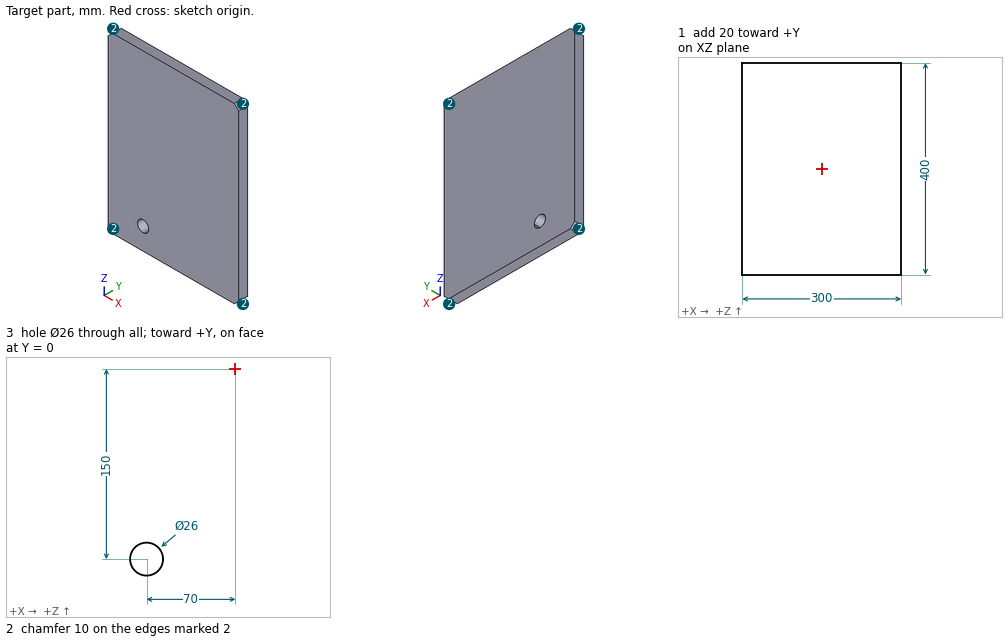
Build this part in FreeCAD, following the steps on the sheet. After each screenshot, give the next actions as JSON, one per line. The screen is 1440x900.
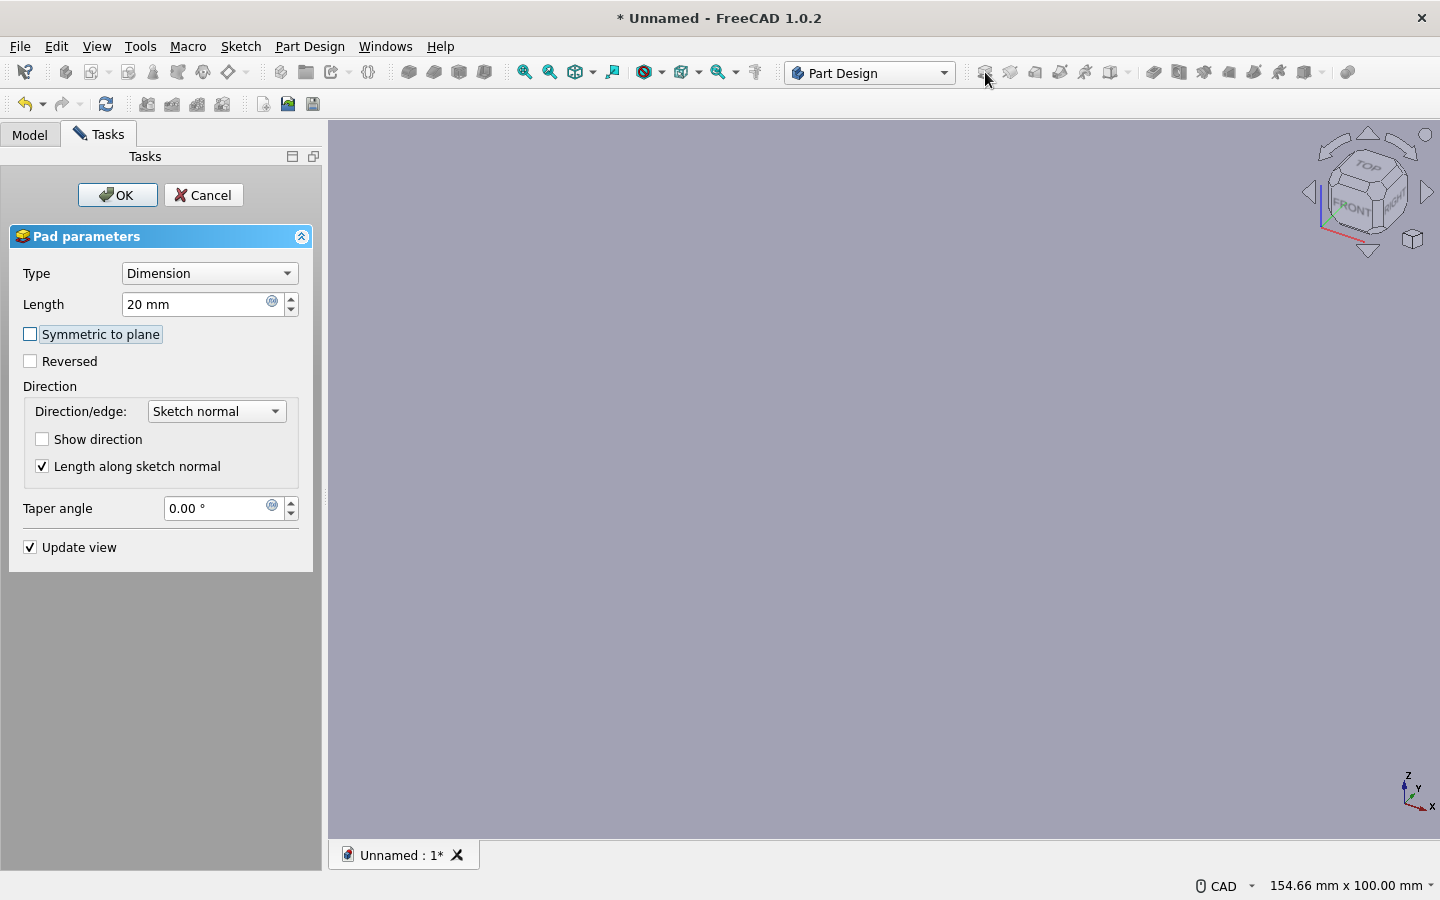
{"action": "left_click", "coordinate": [31, 361]}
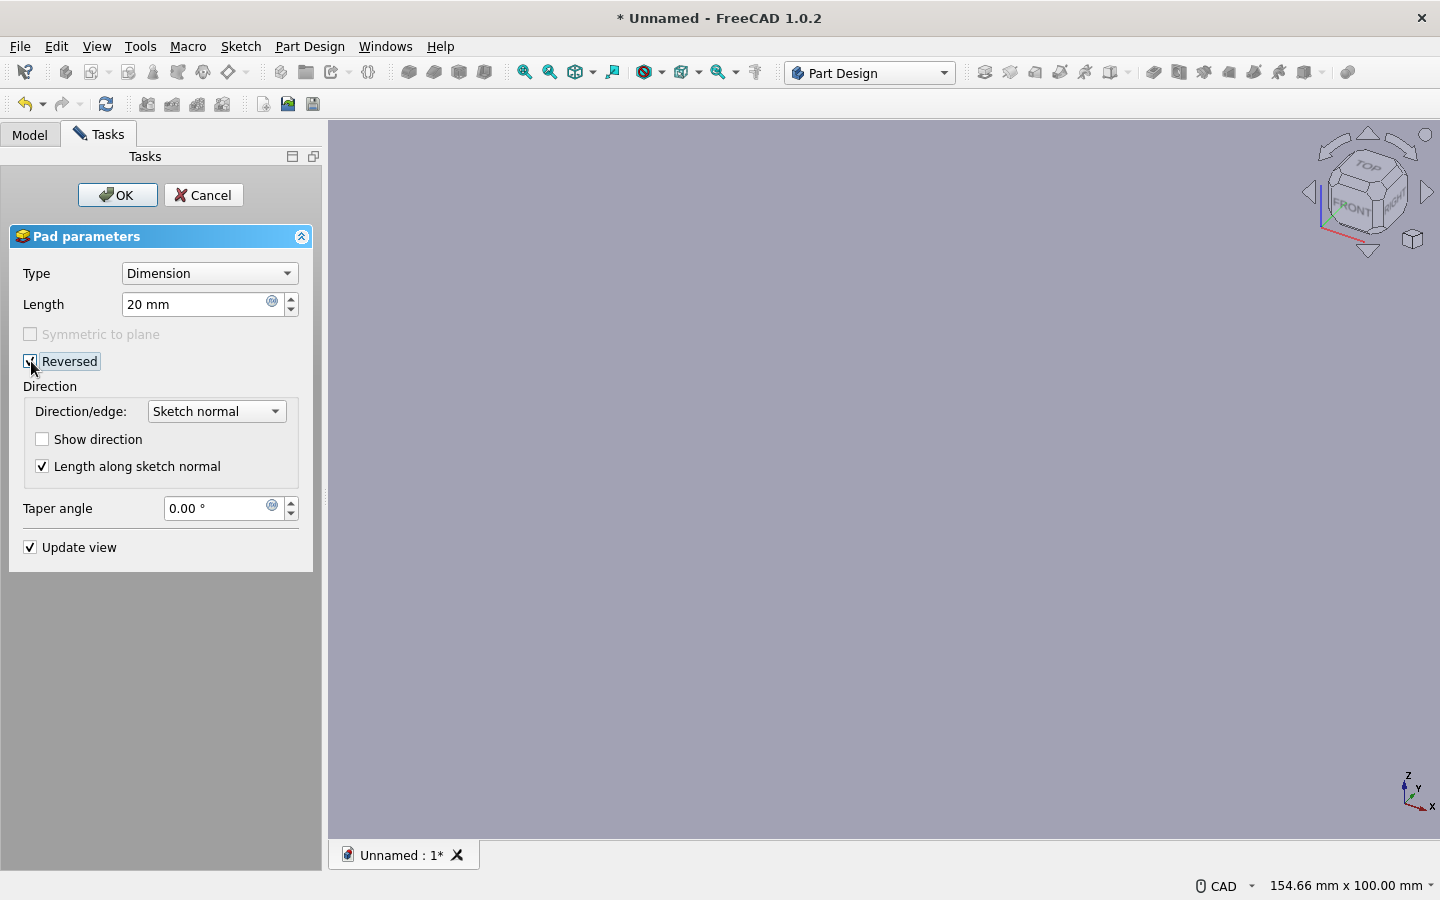
{"action": "left_click", "coordinate": [118, 195]}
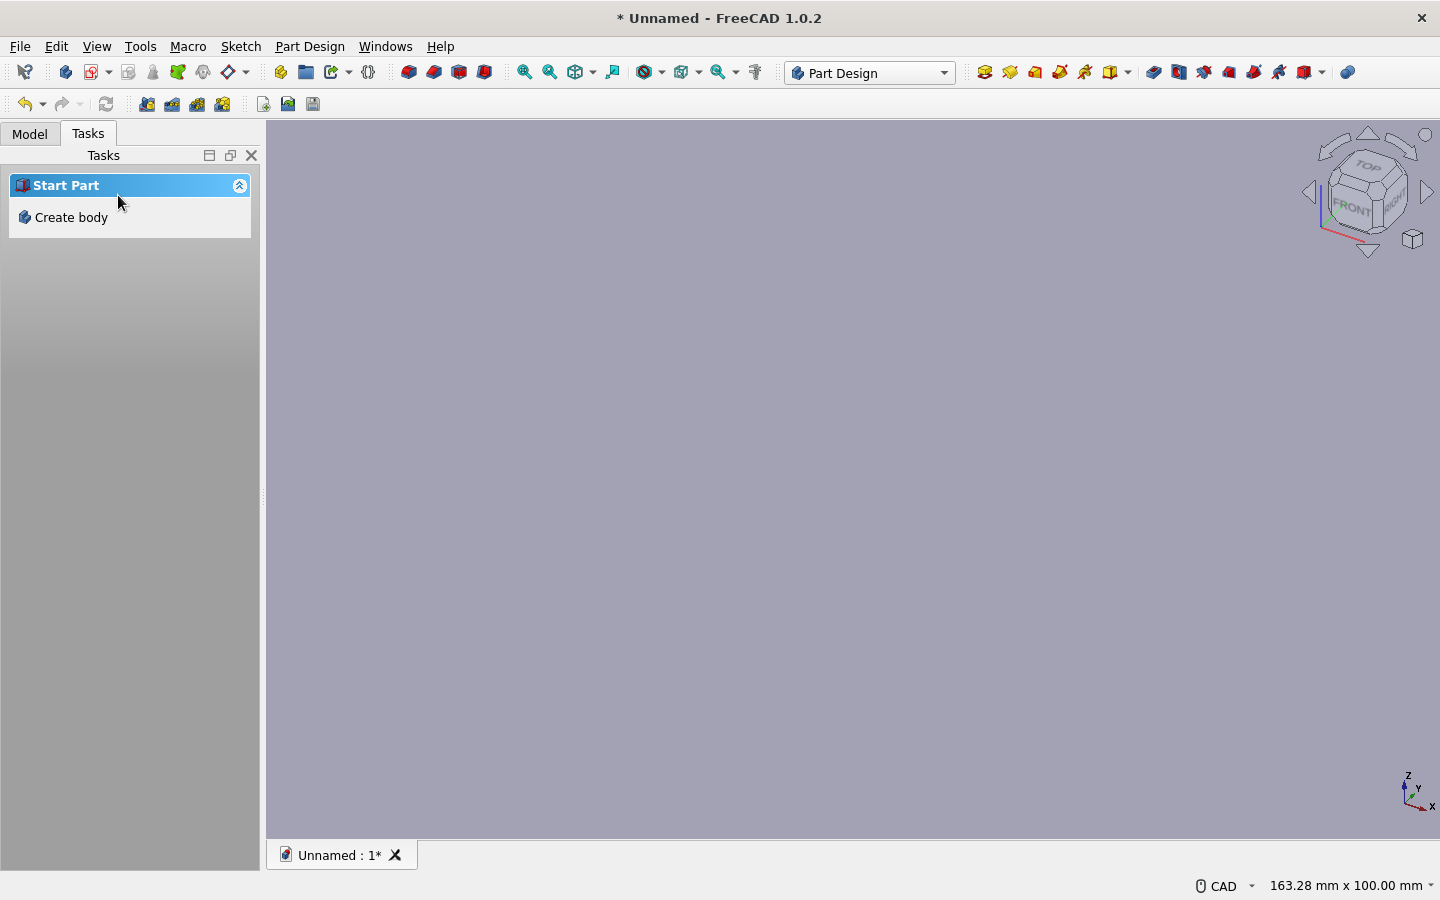
{"action": "left_click", "coordinate": [525, 72]}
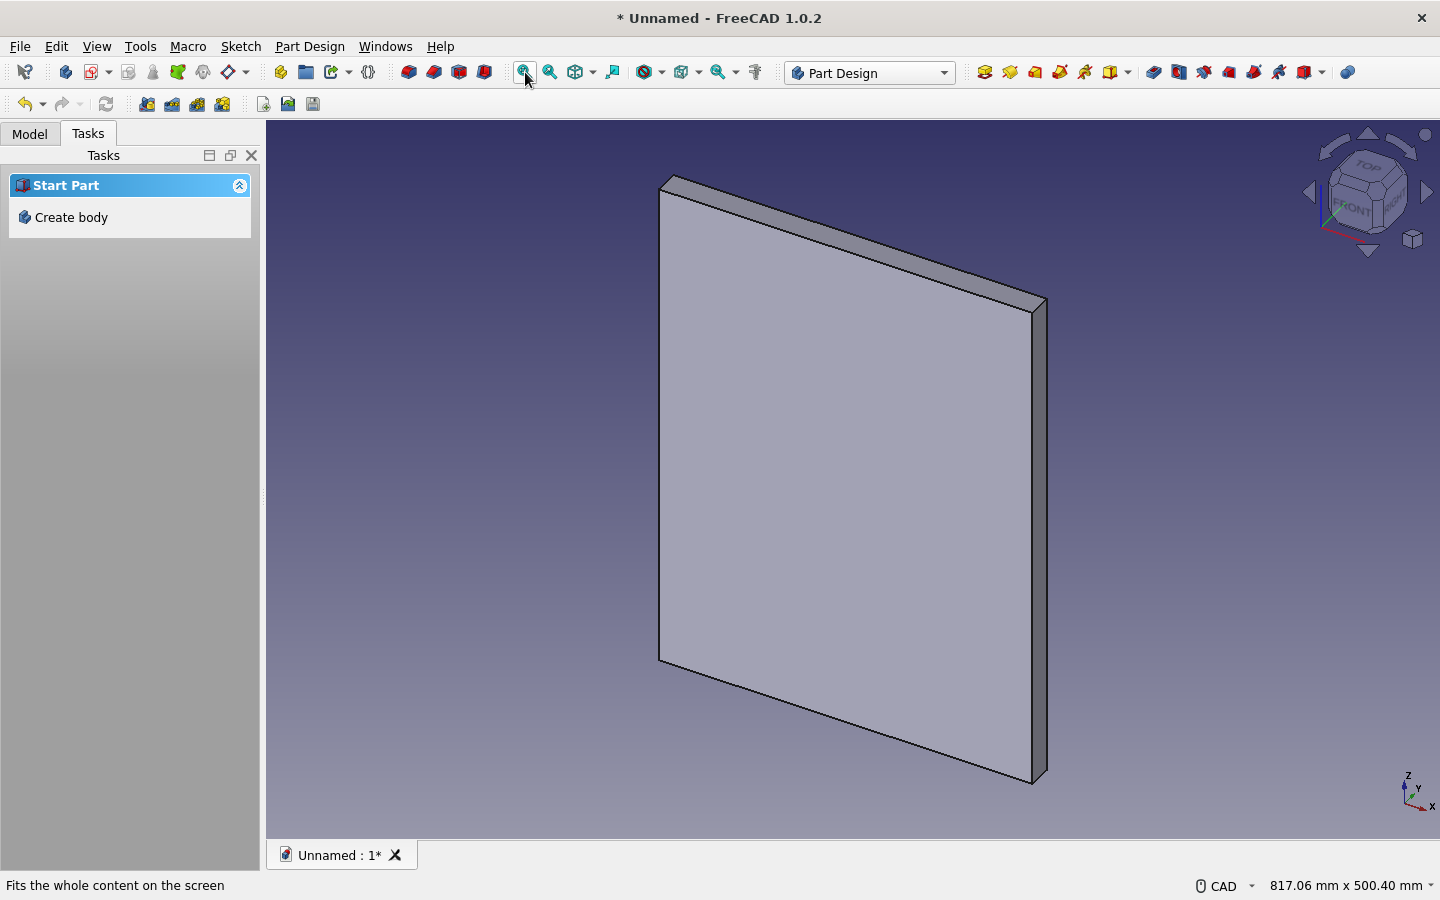
{"action": "left_click", "coordinate": [1040, 305]}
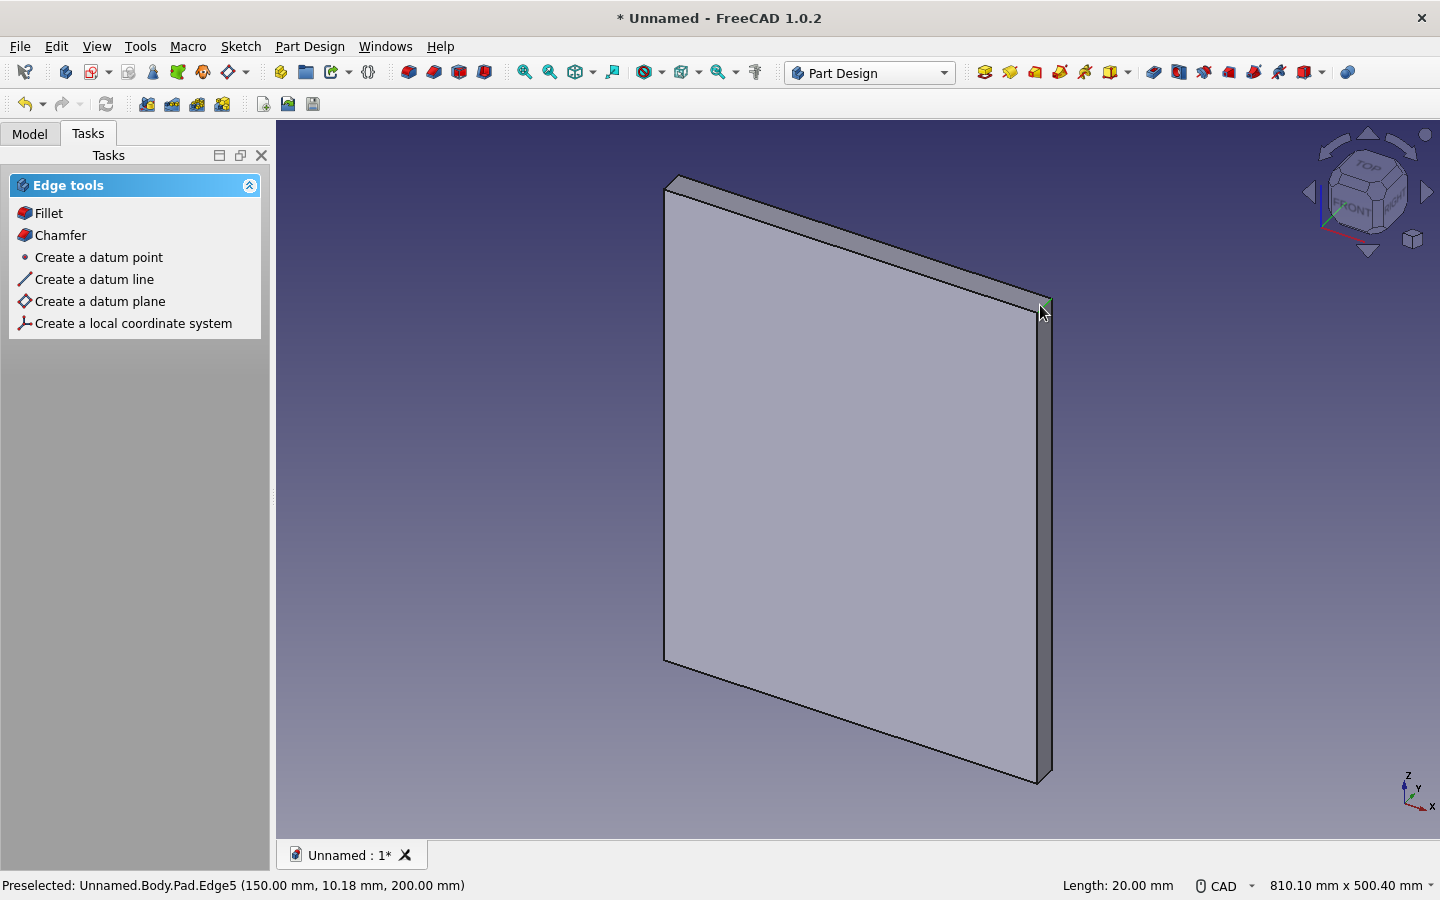
{"action": "key", "text": "0"}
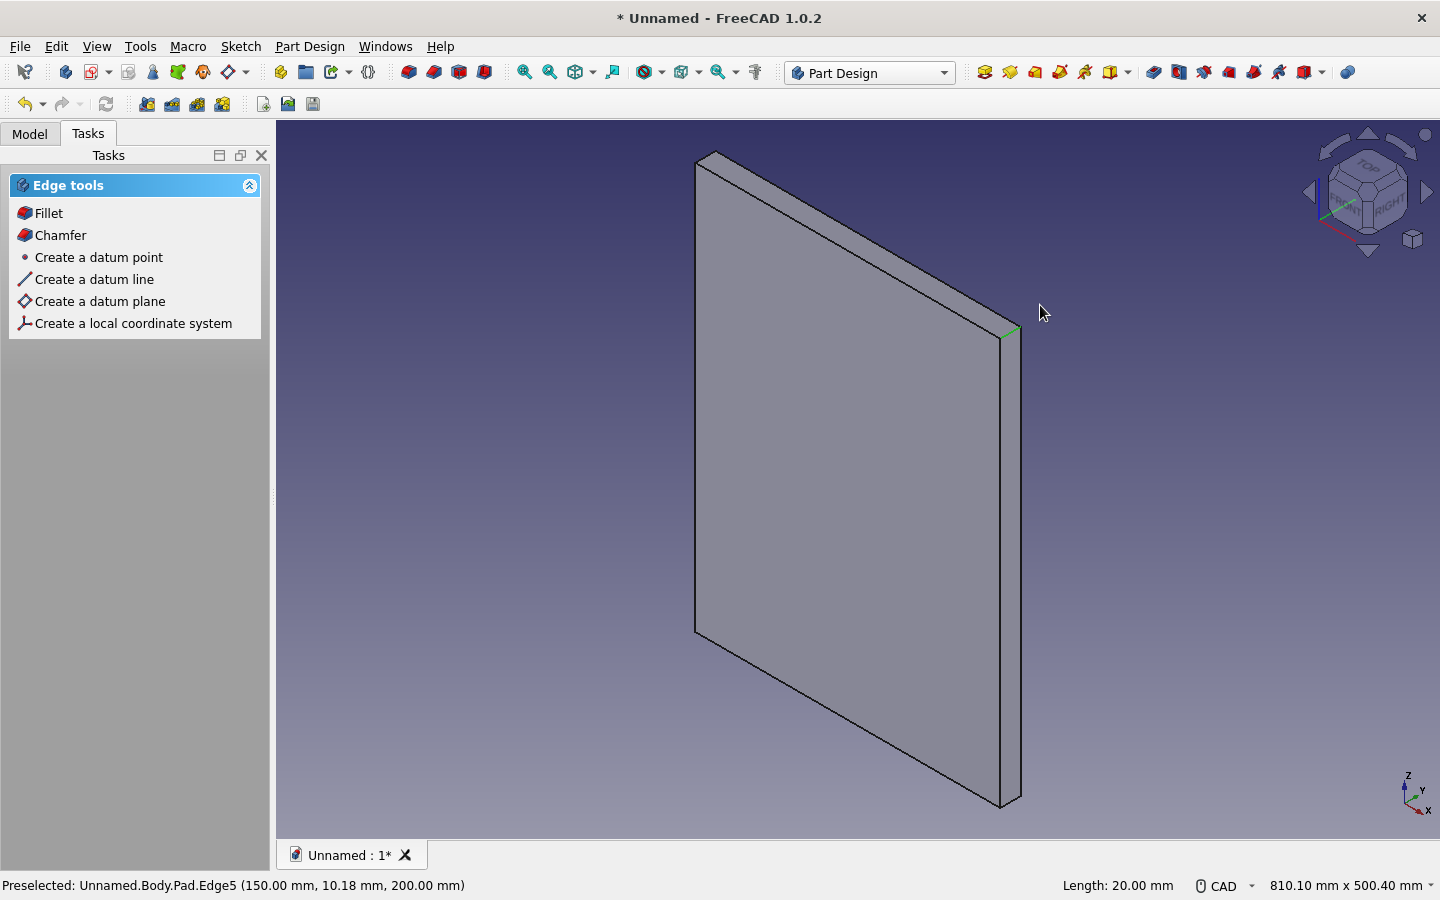
{"action": "key", "text": "2"}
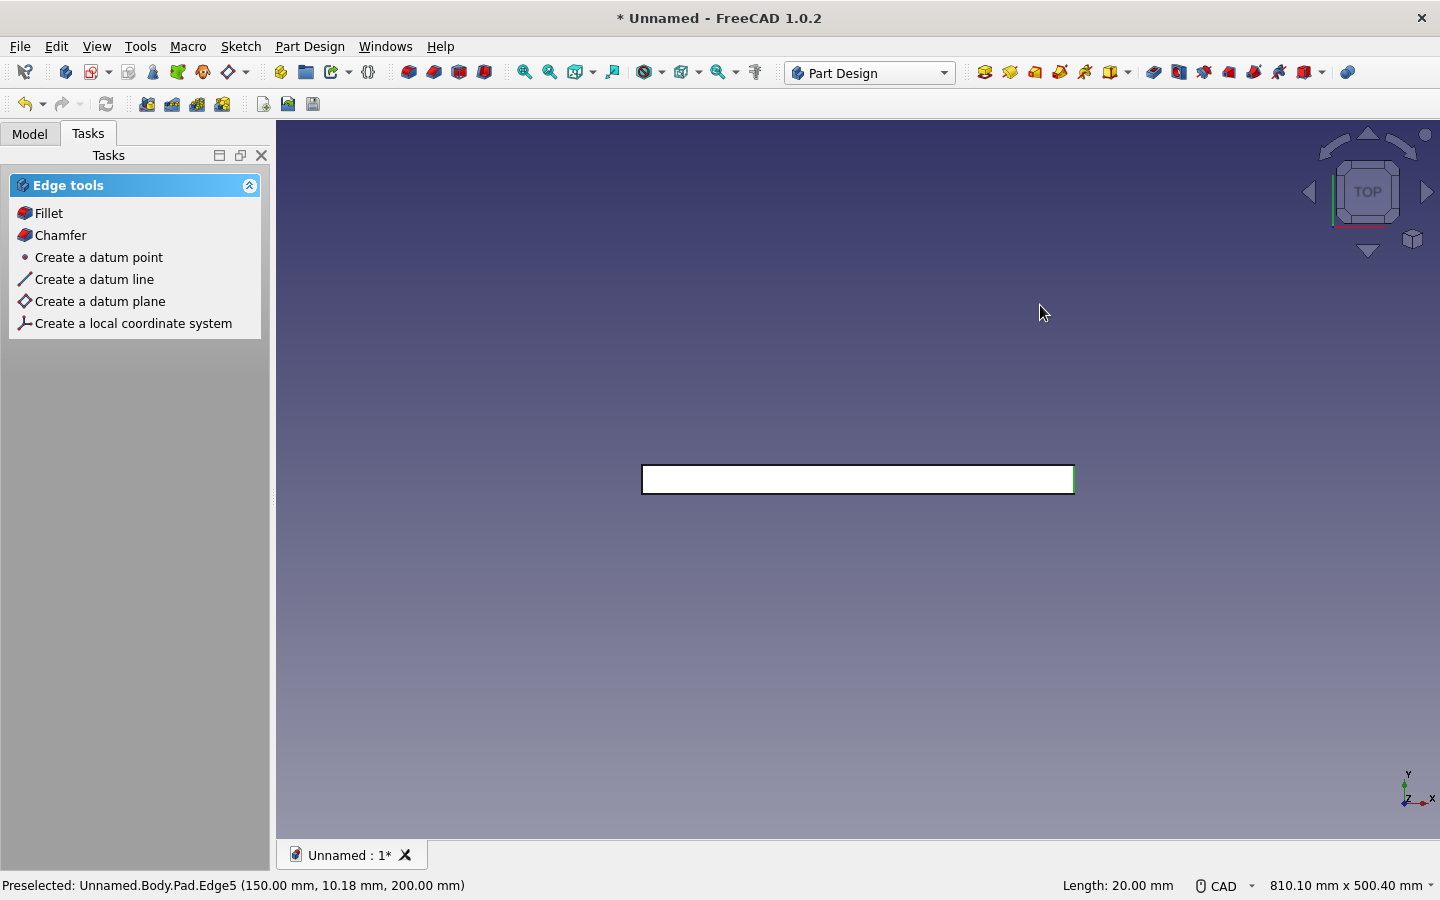
{"action": "left_click", "coordinate": [525, 72]}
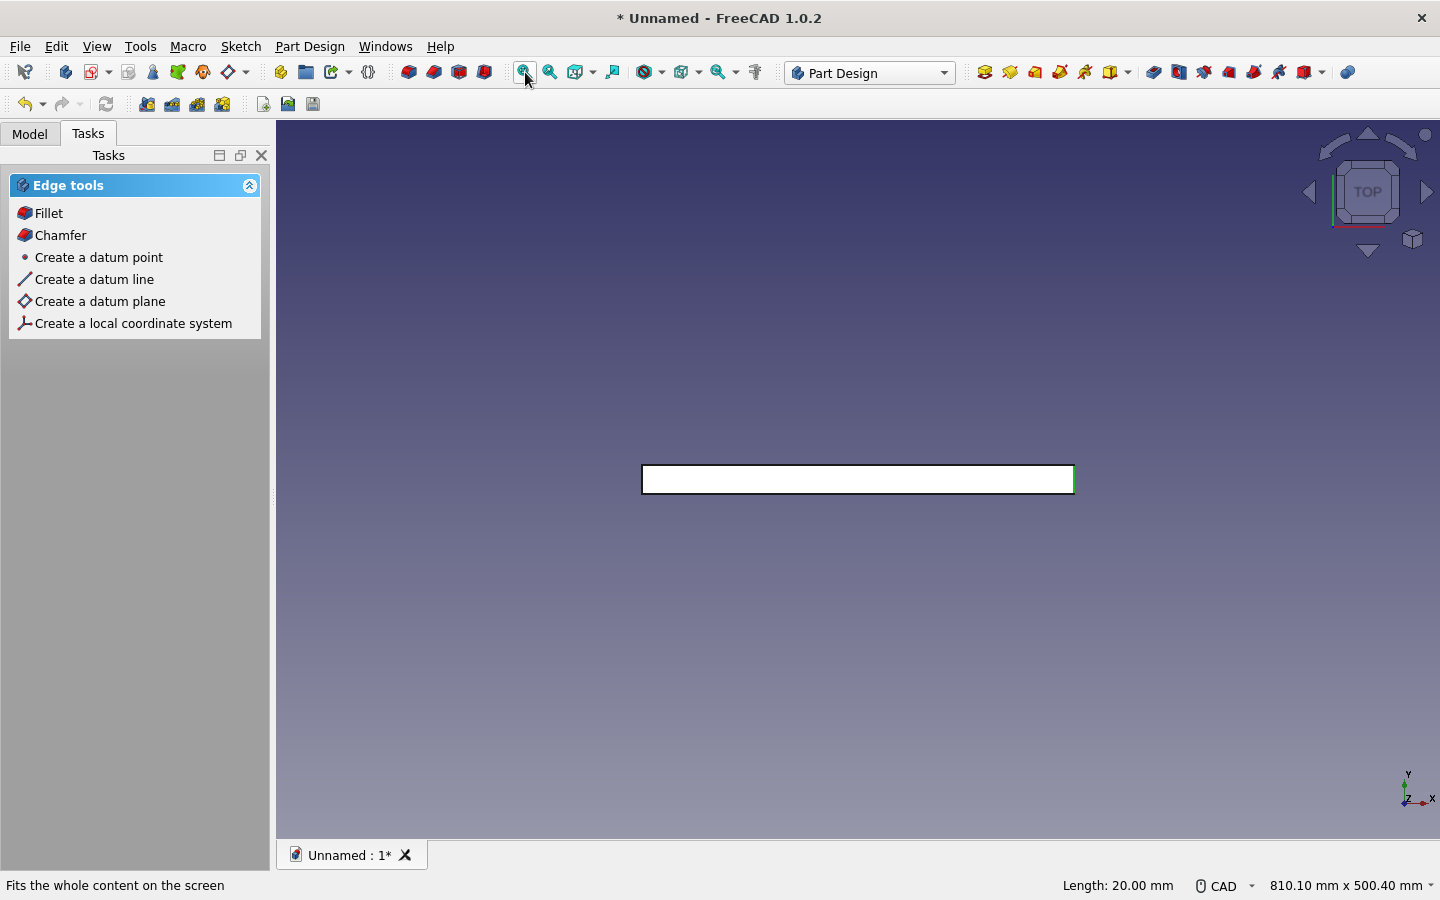
{"action": "left_click", "coordinate": [642, 478], "text": "ctrl"}